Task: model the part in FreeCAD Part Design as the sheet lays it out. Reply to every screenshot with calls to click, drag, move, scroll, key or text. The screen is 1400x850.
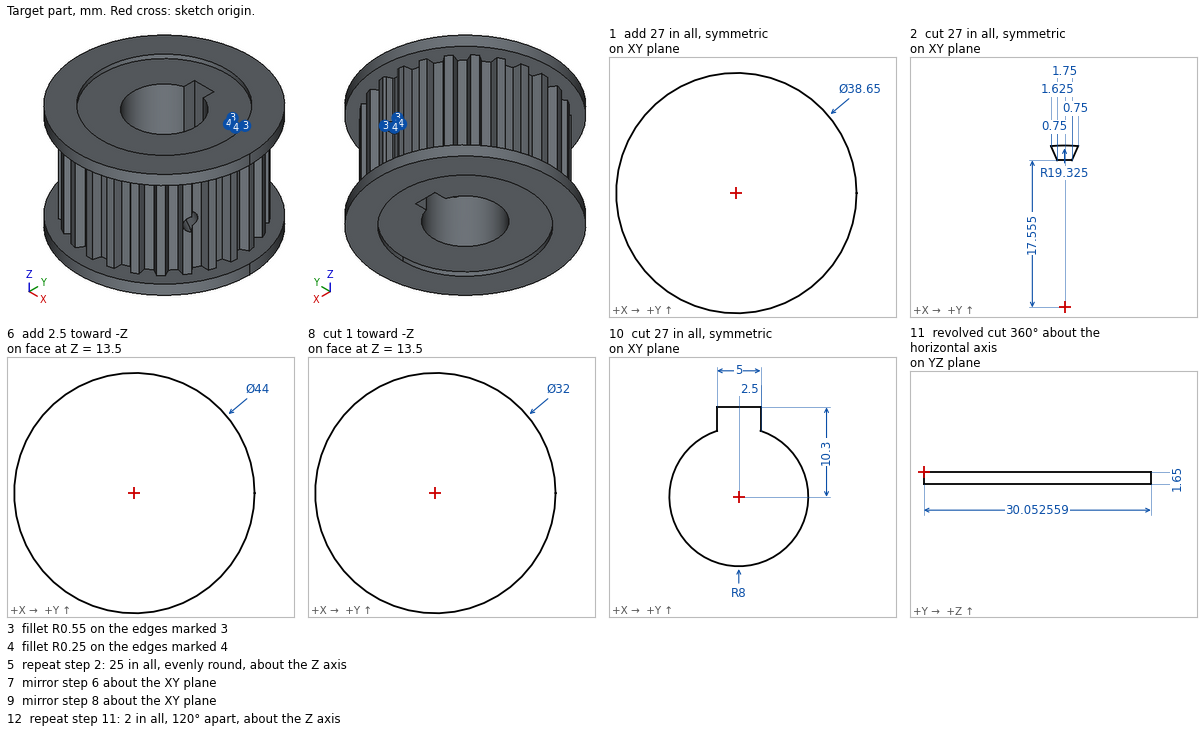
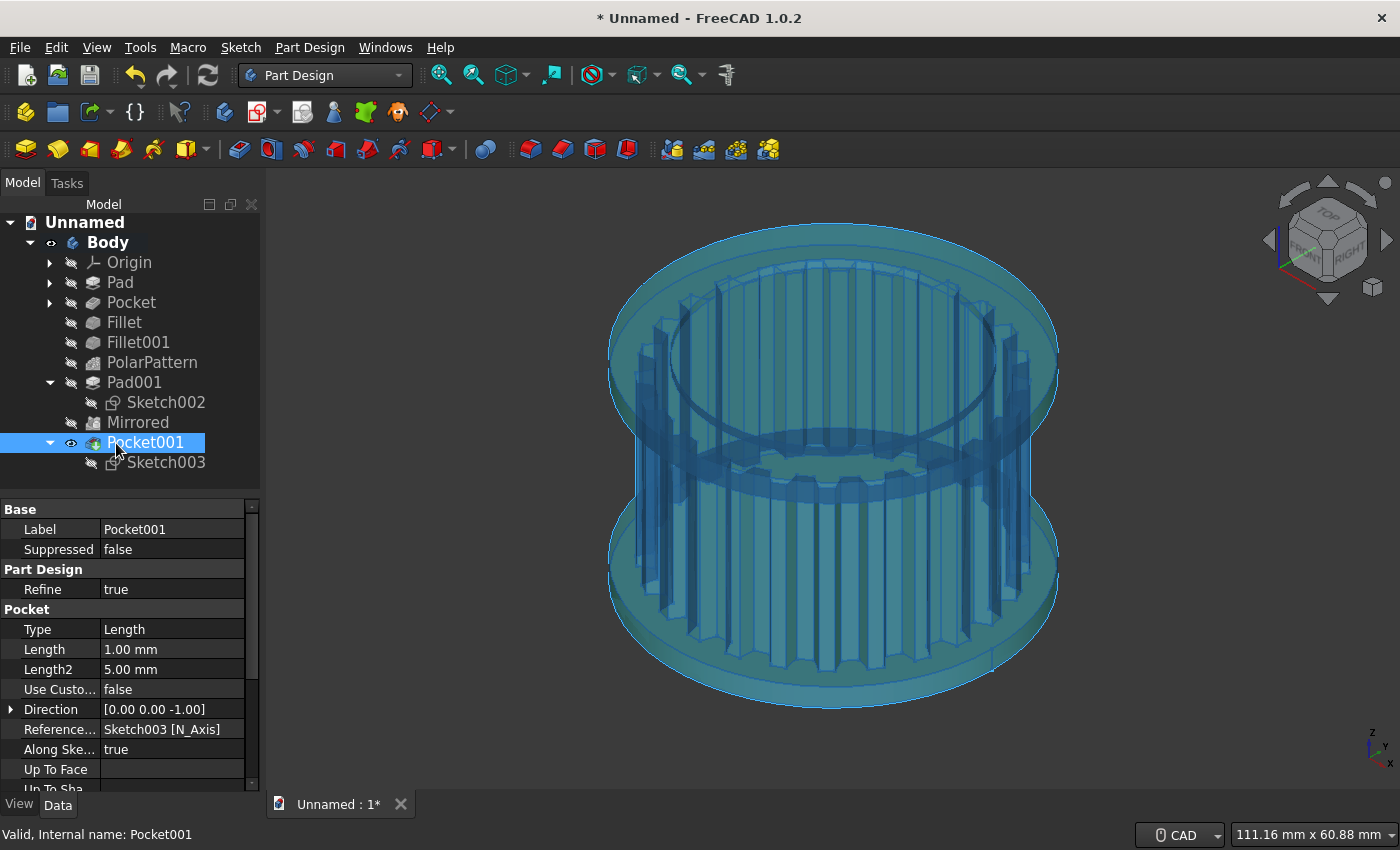
click(672, 150)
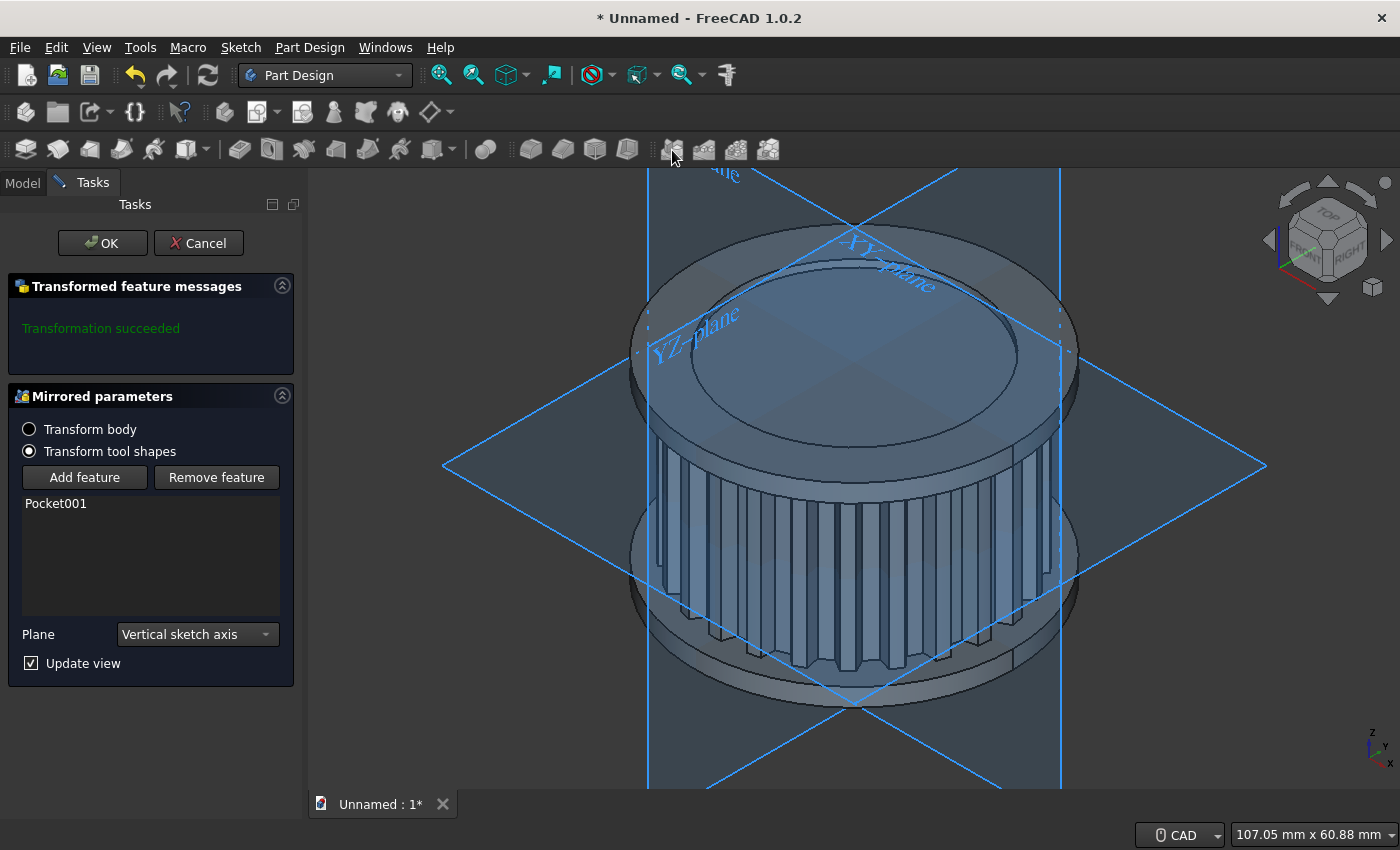
click(198, 634)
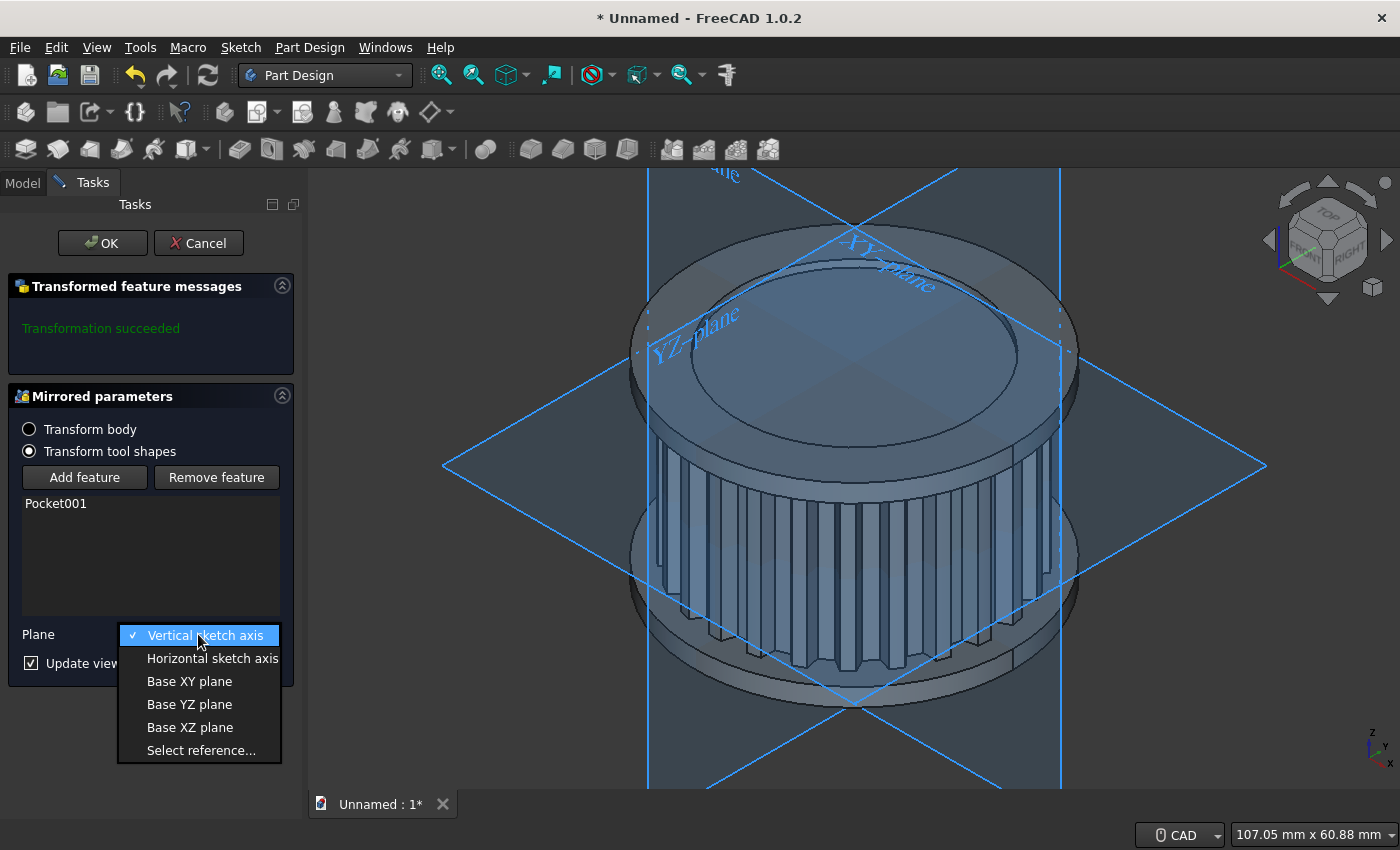
click(198, 682)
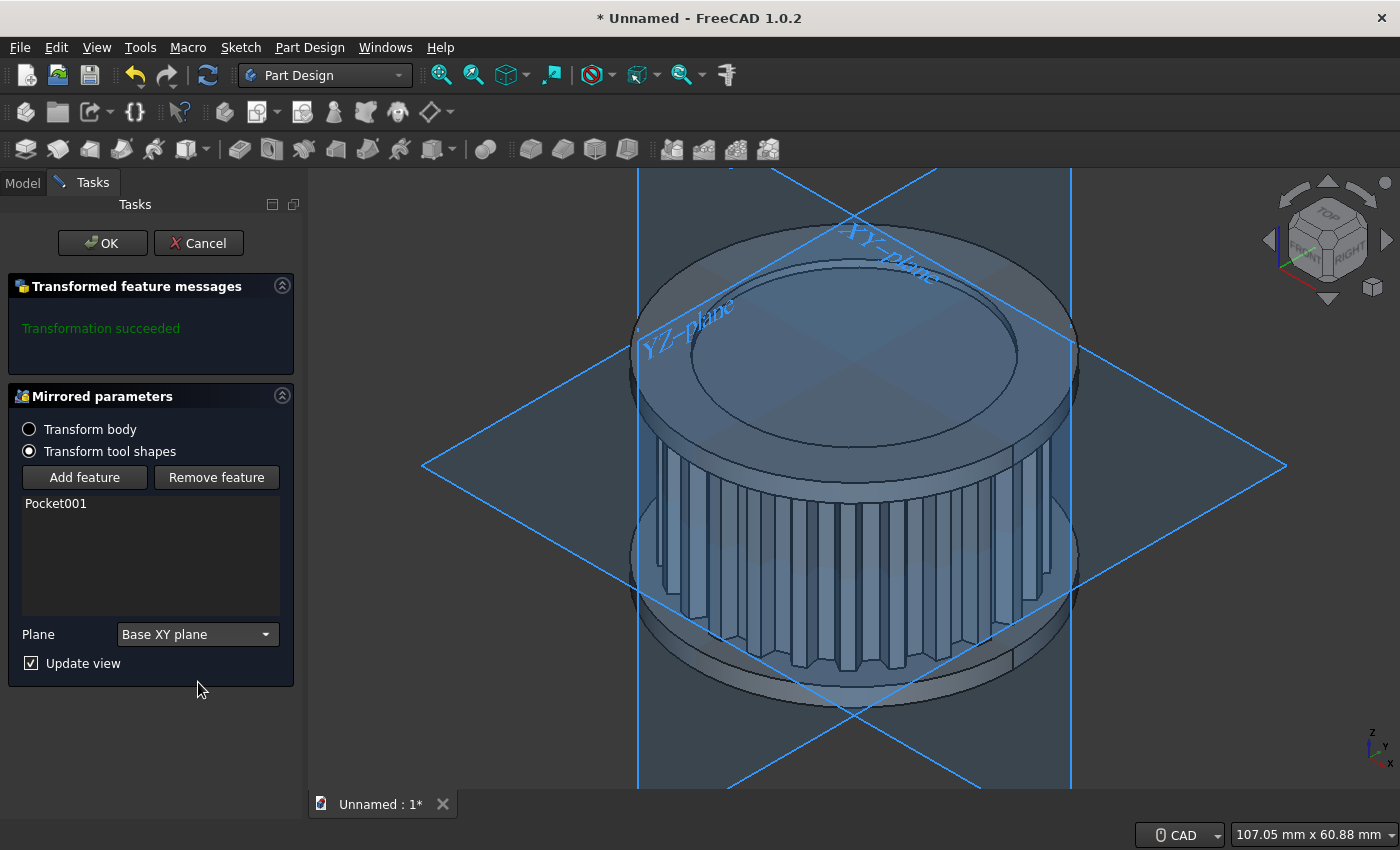
click(103, 243)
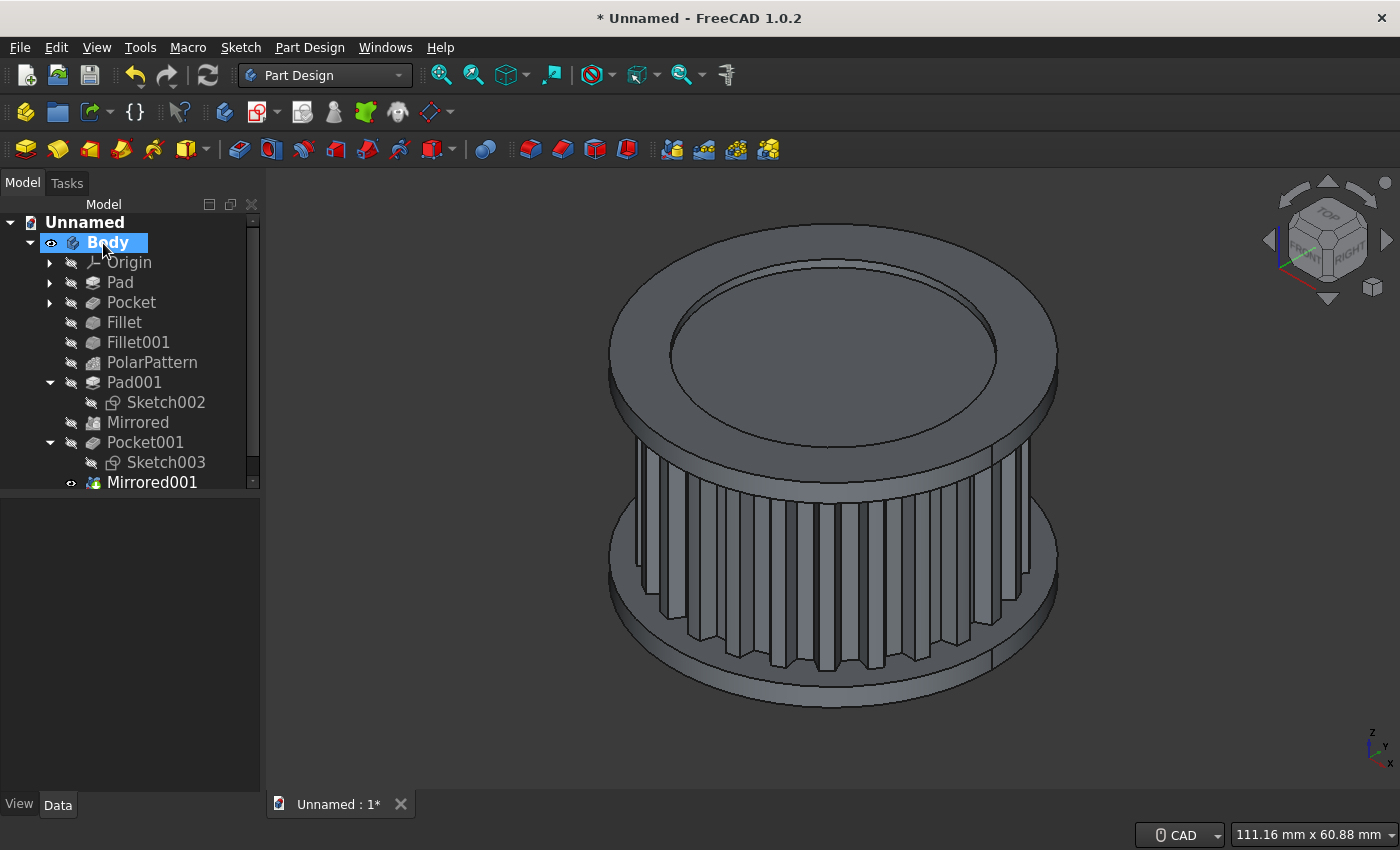
click(258, 112)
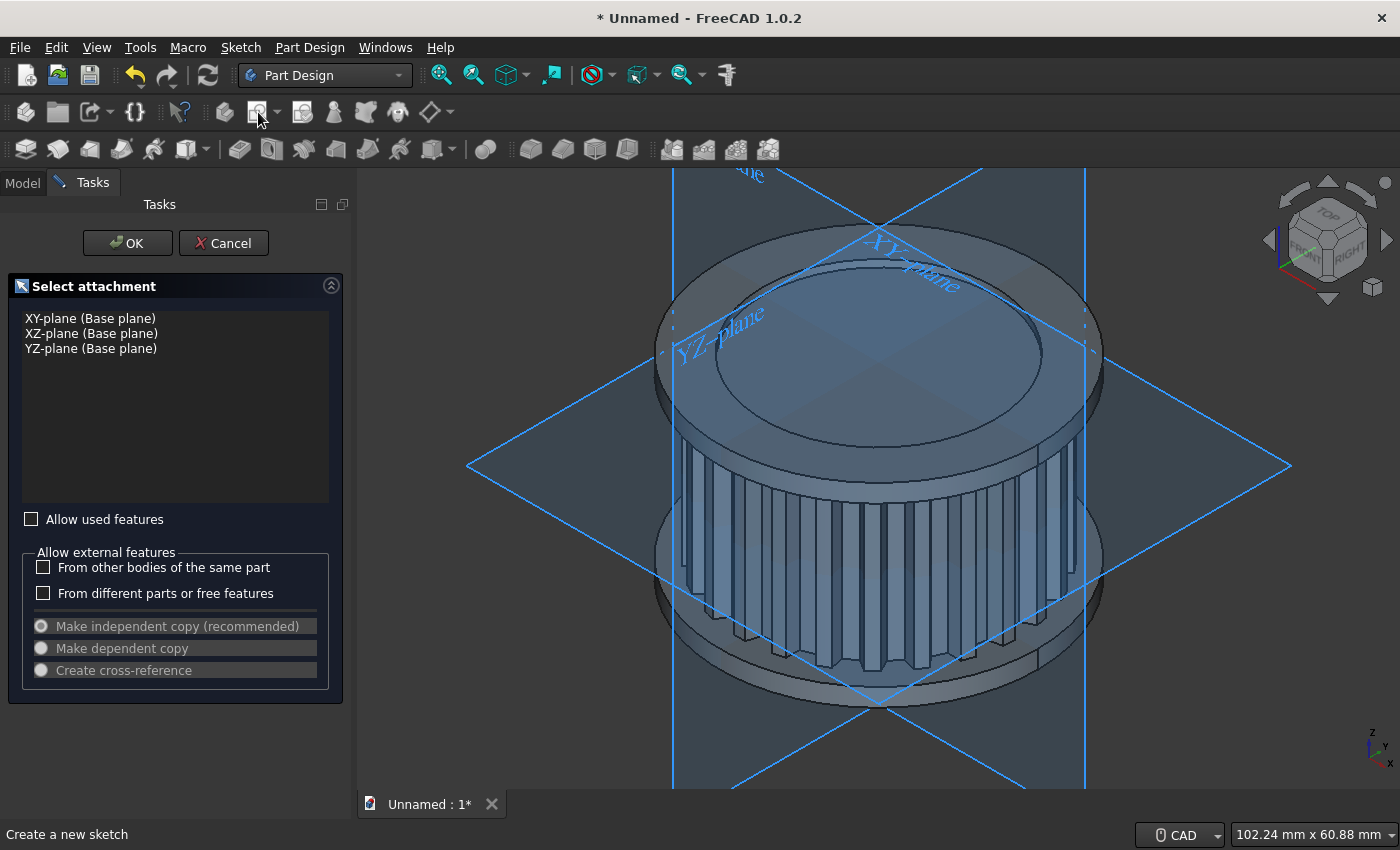
click(82, 318)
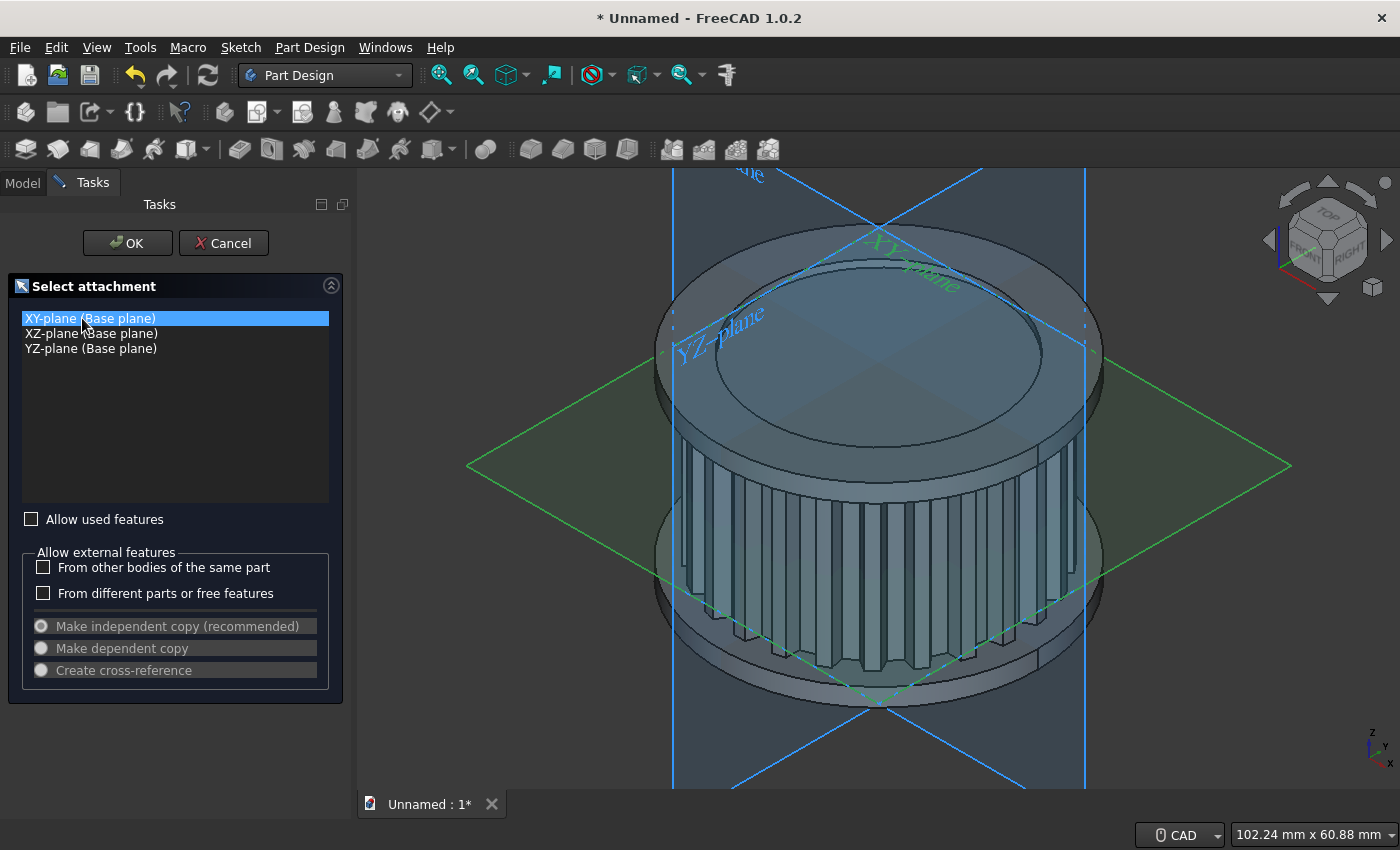
click(128, 243)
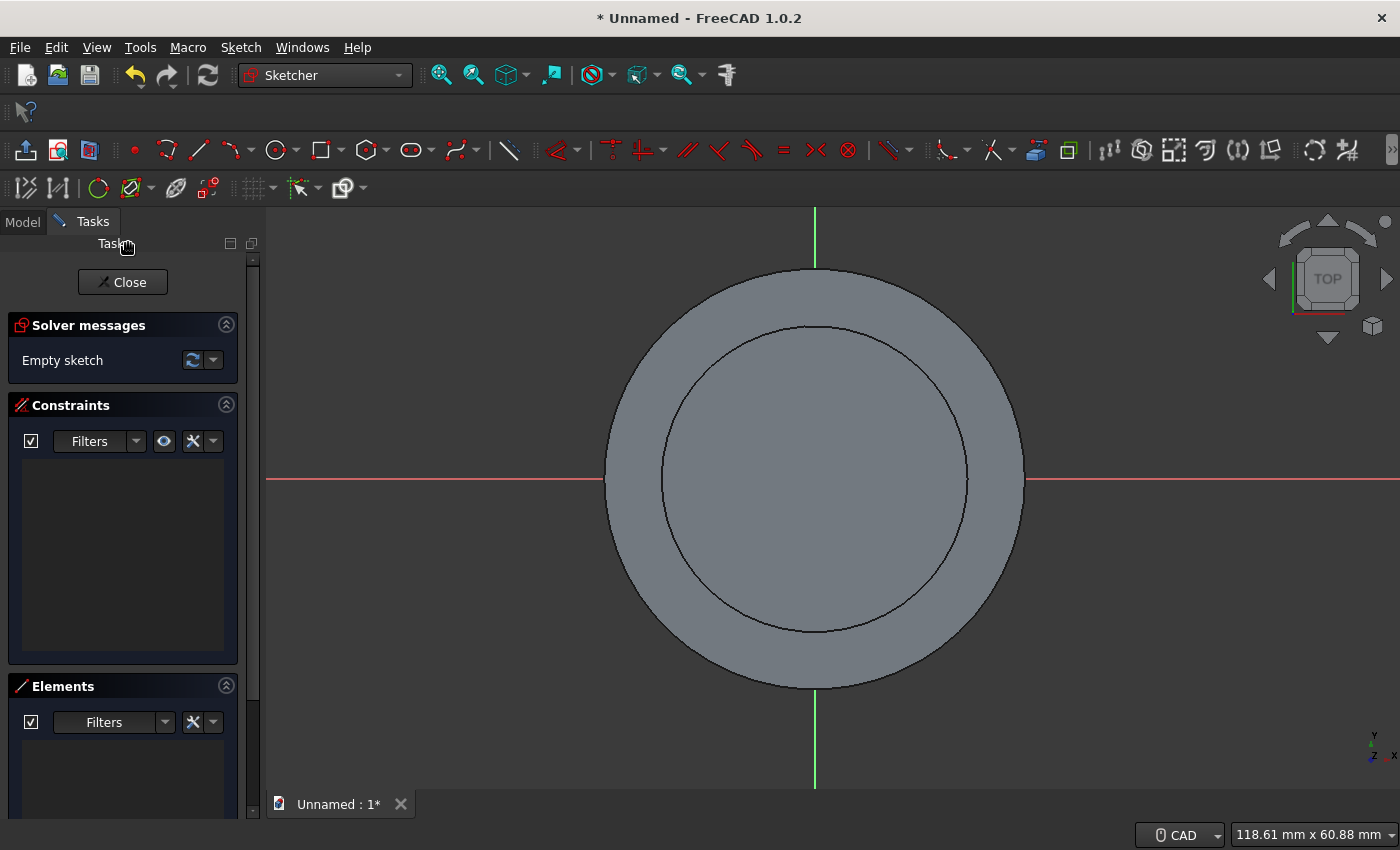
click(90, 150)